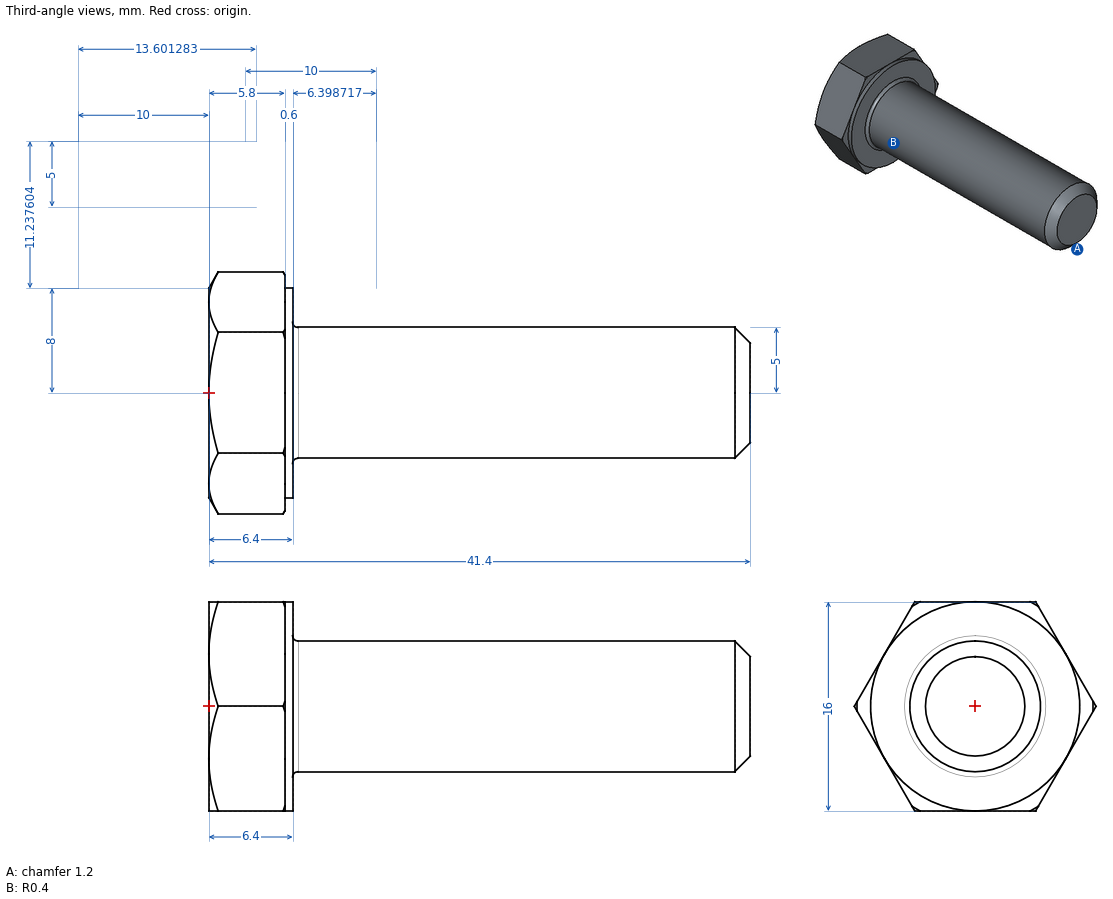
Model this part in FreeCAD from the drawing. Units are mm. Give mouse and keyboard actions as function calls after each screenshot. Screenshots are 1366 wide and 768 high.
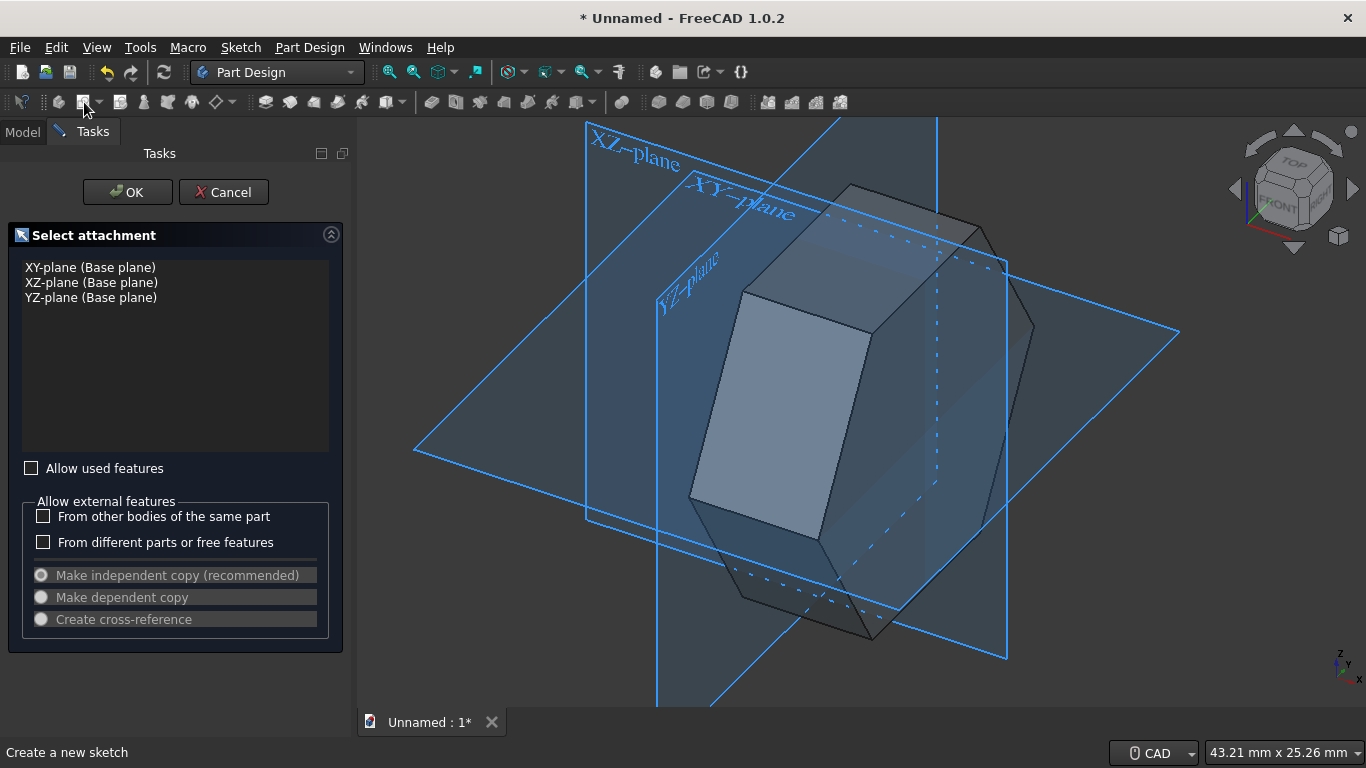
click(82, 268)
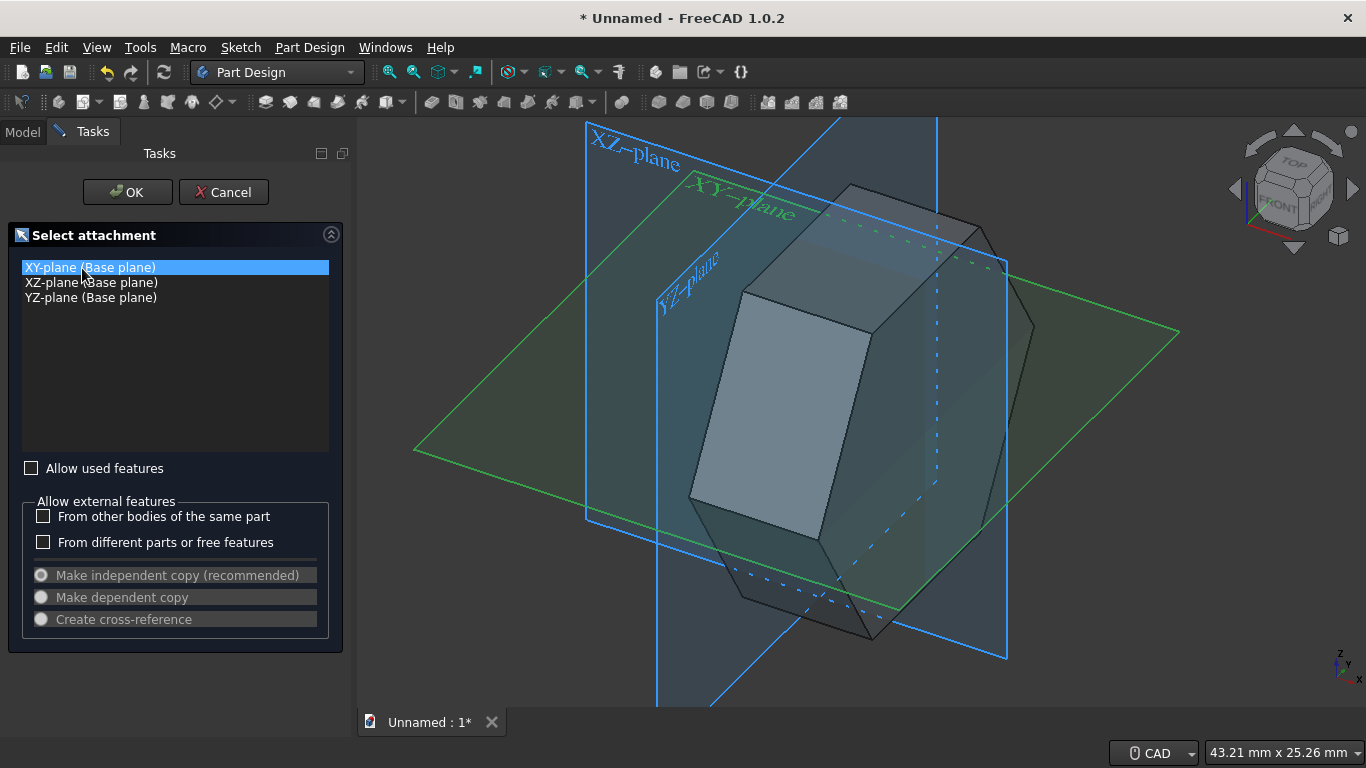
click(128, 192)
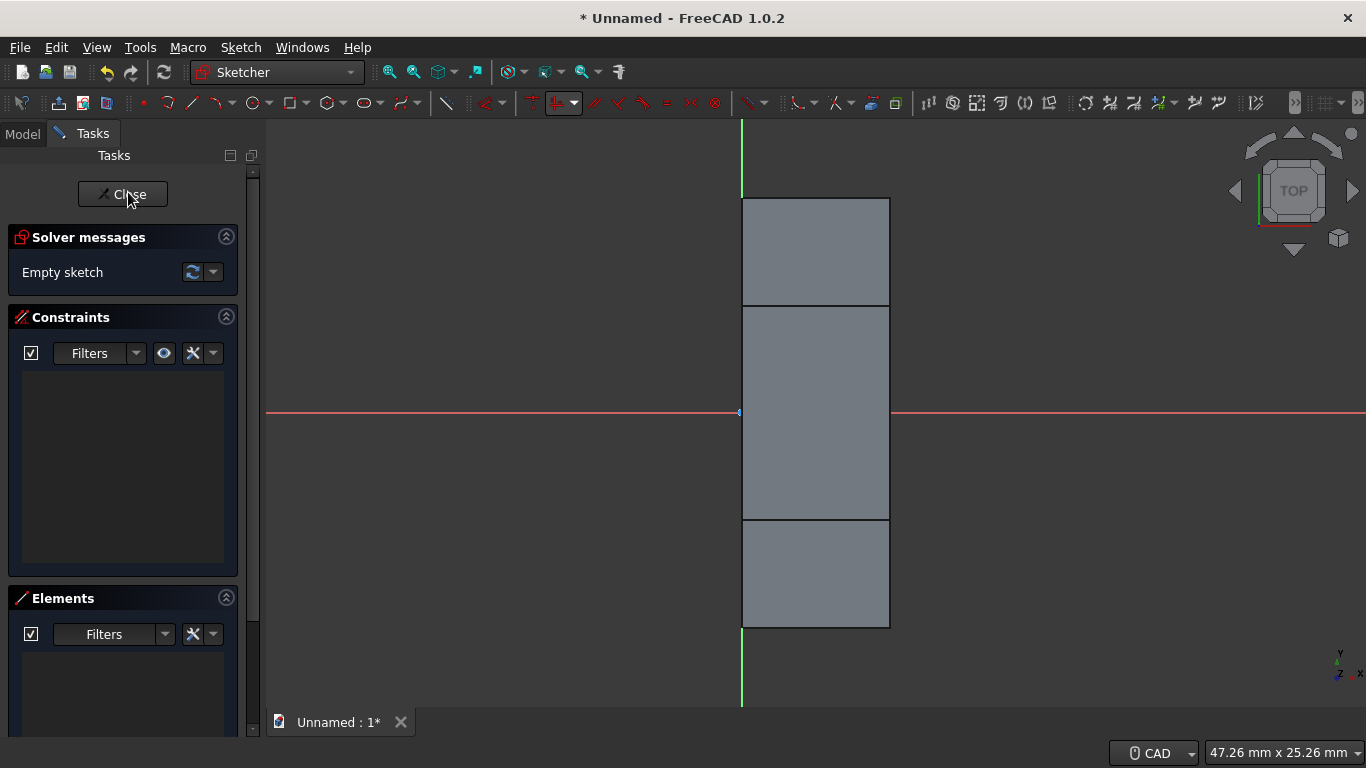
click(108, 104)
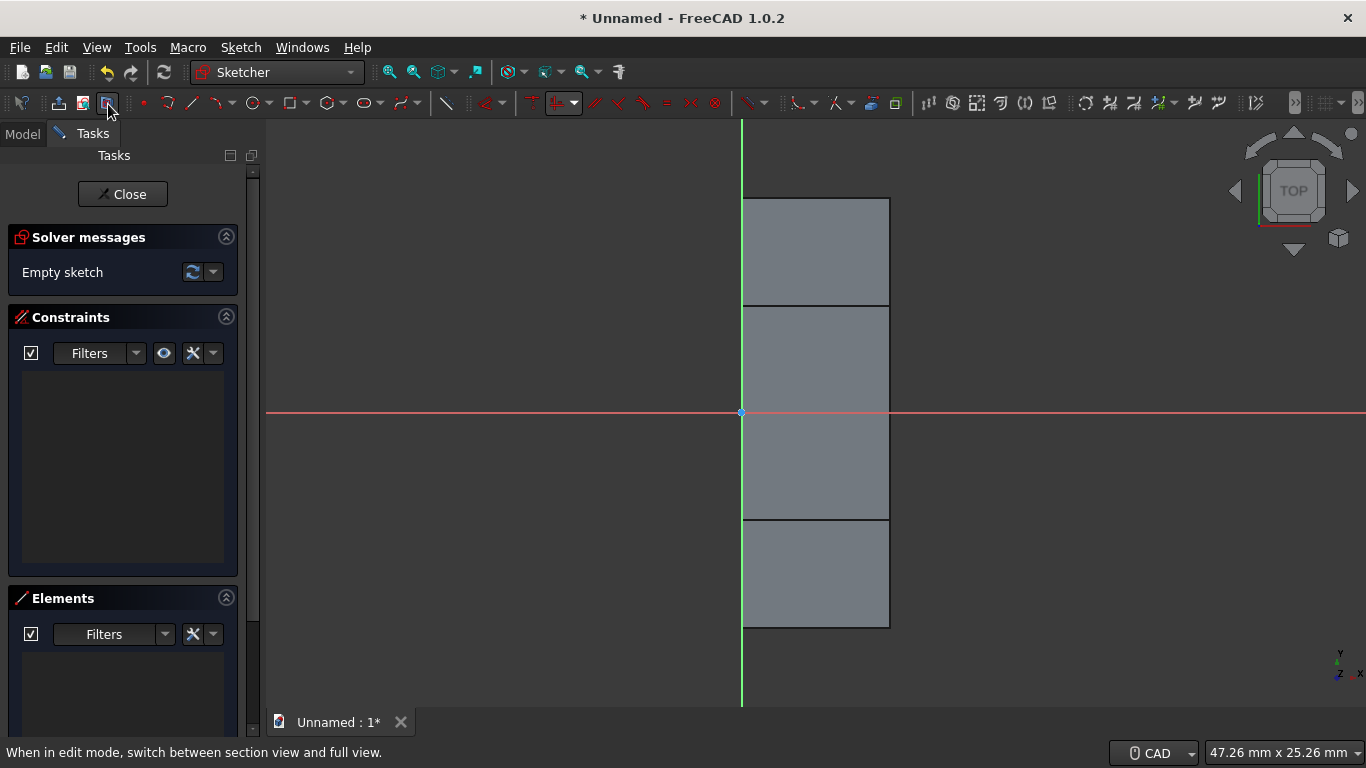
scroll(294, 484, down, 3)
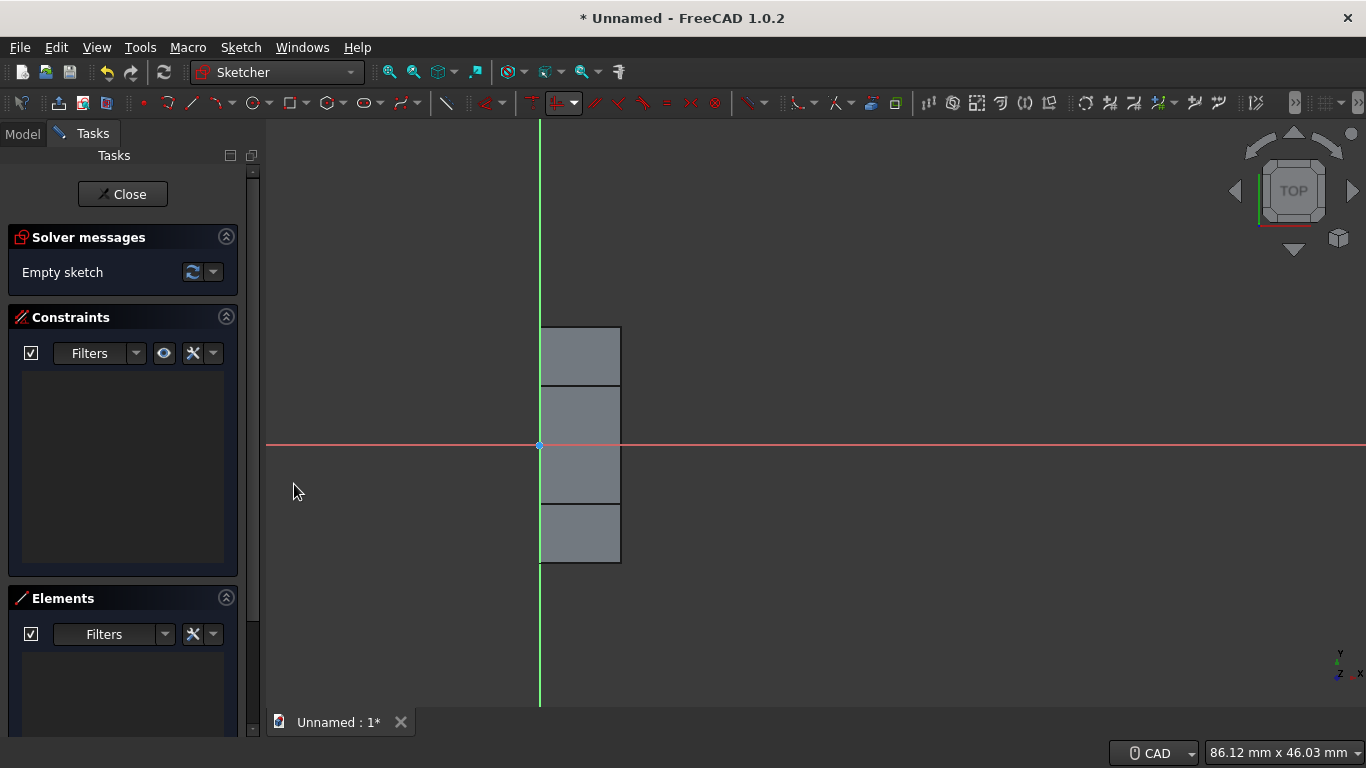
click(290, 104)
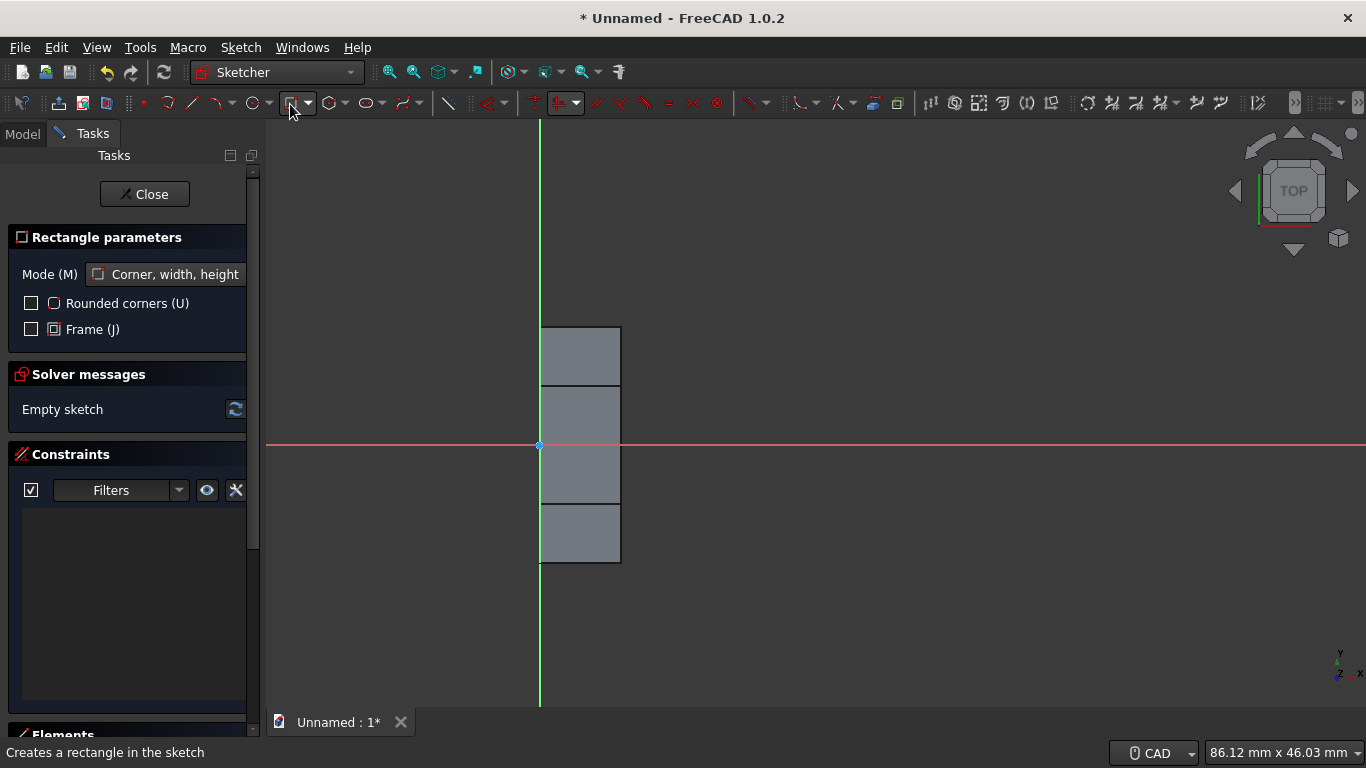
click(540, 445)
move(1068, 381)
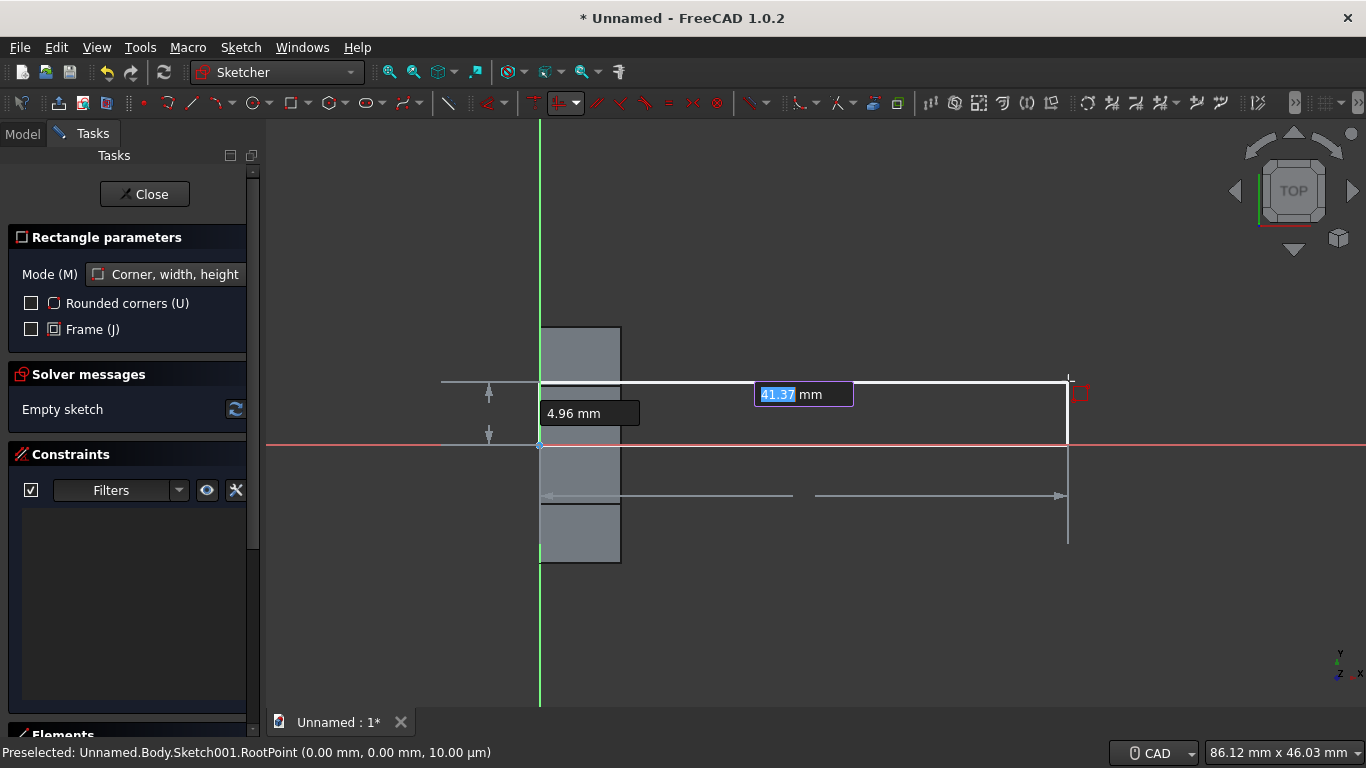
text(41.4)
key(Tab)
text(5)
key(Return)
key(Escape)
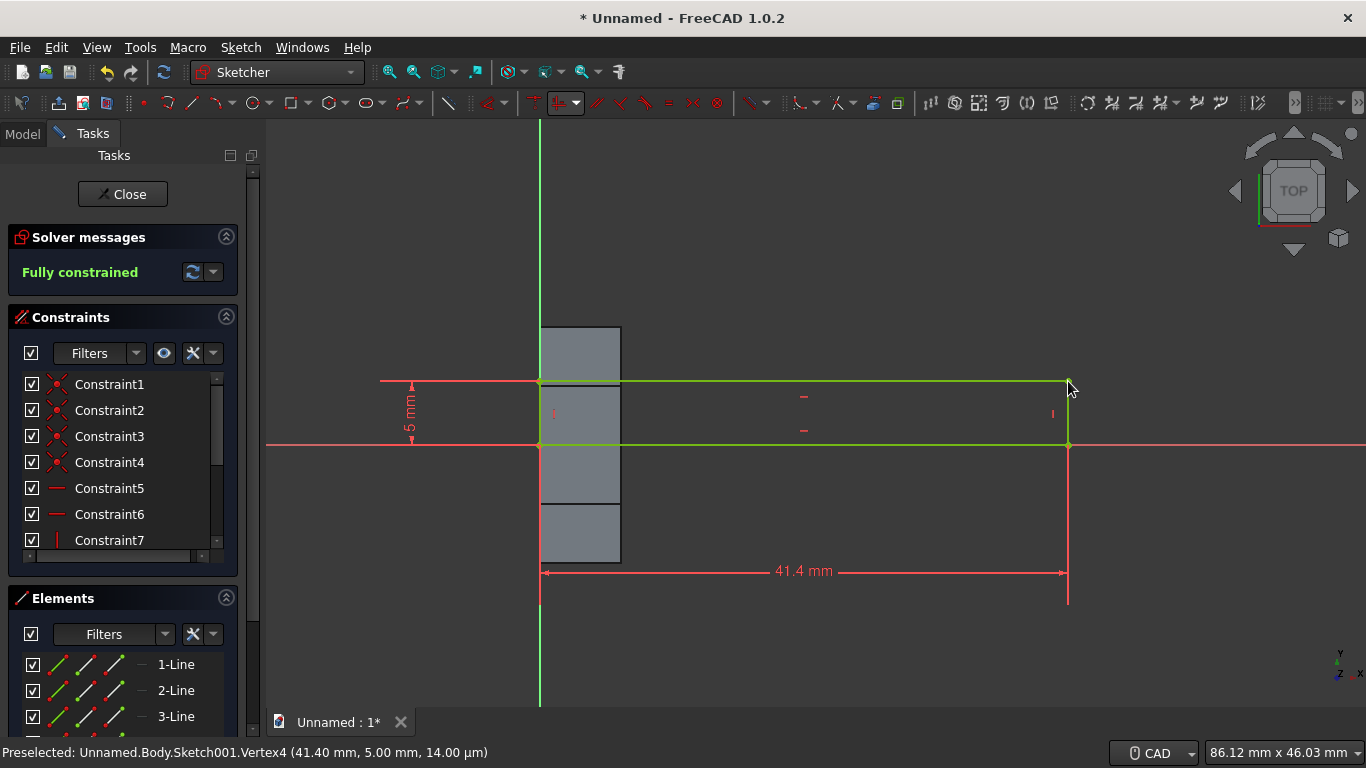
click(123, 194)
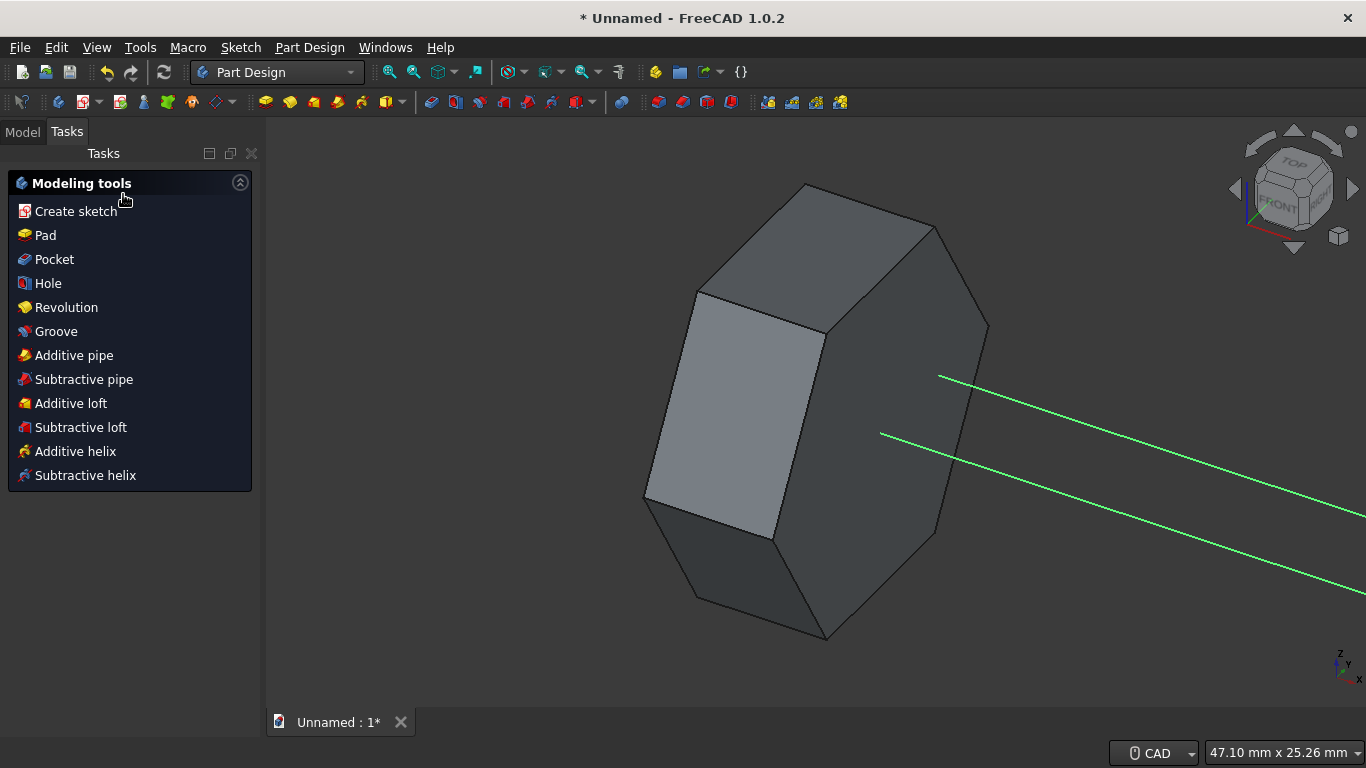
click(290, 102)